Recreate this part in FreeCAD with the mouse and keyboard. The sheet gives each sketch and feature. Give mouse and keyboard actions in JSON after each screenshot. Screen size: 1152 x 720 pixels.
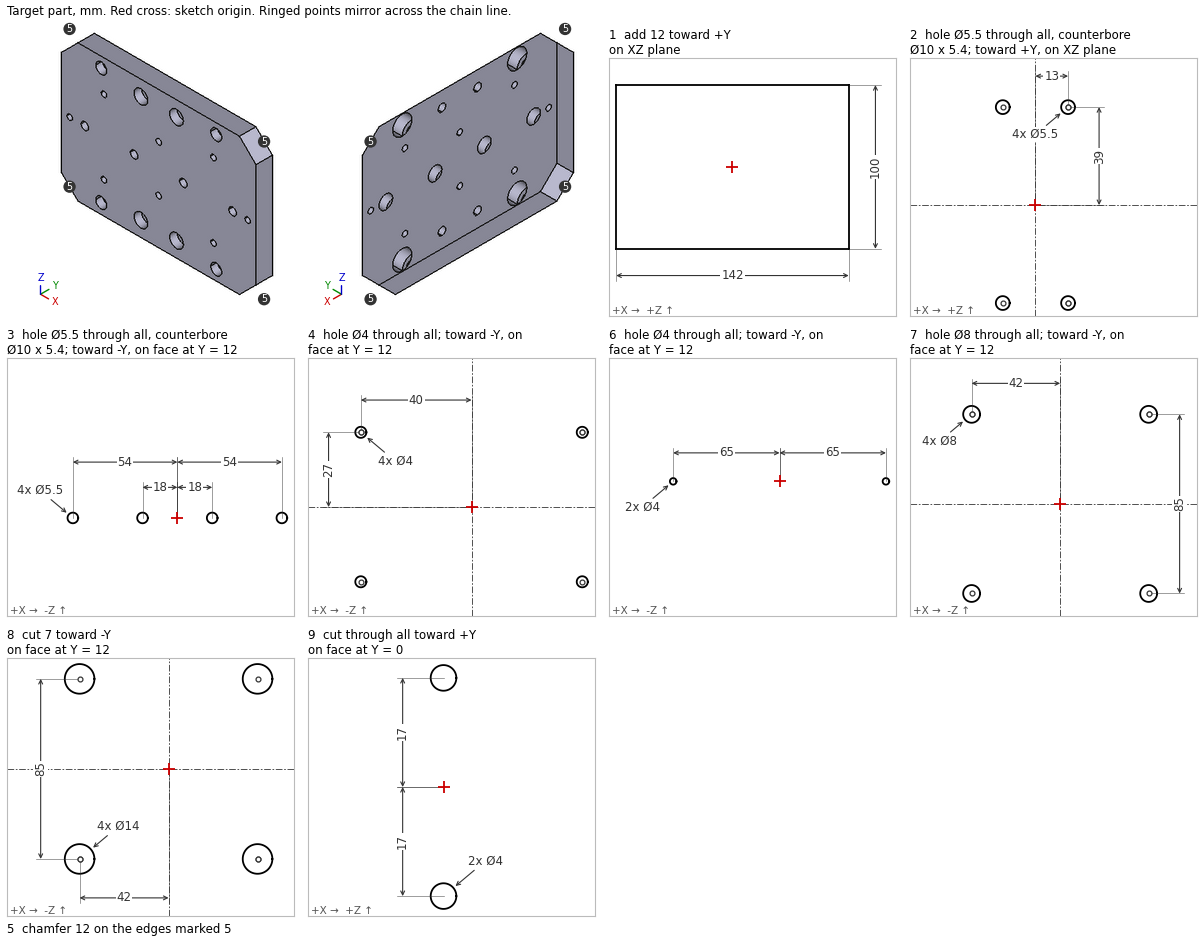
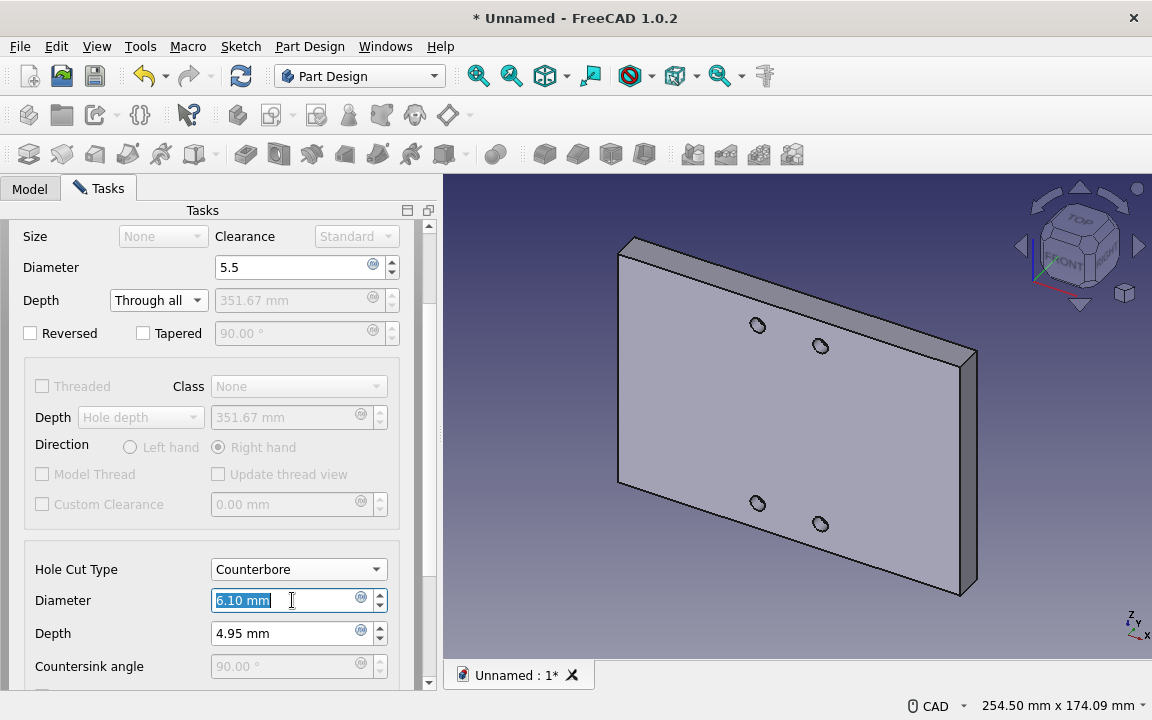
{"action": "type", "text": "10"}
{"action": "key", "text": "Tab"}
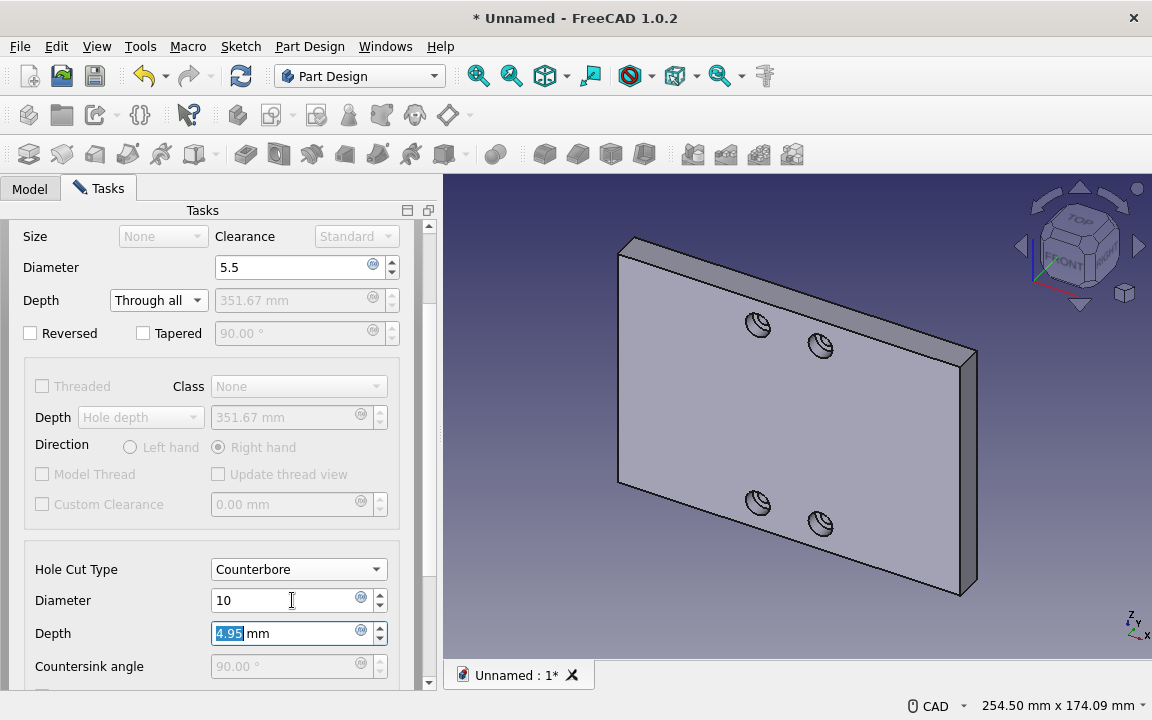
{"action": "type", "text": "5.4"}
{"action": "key", "text": "Tab"}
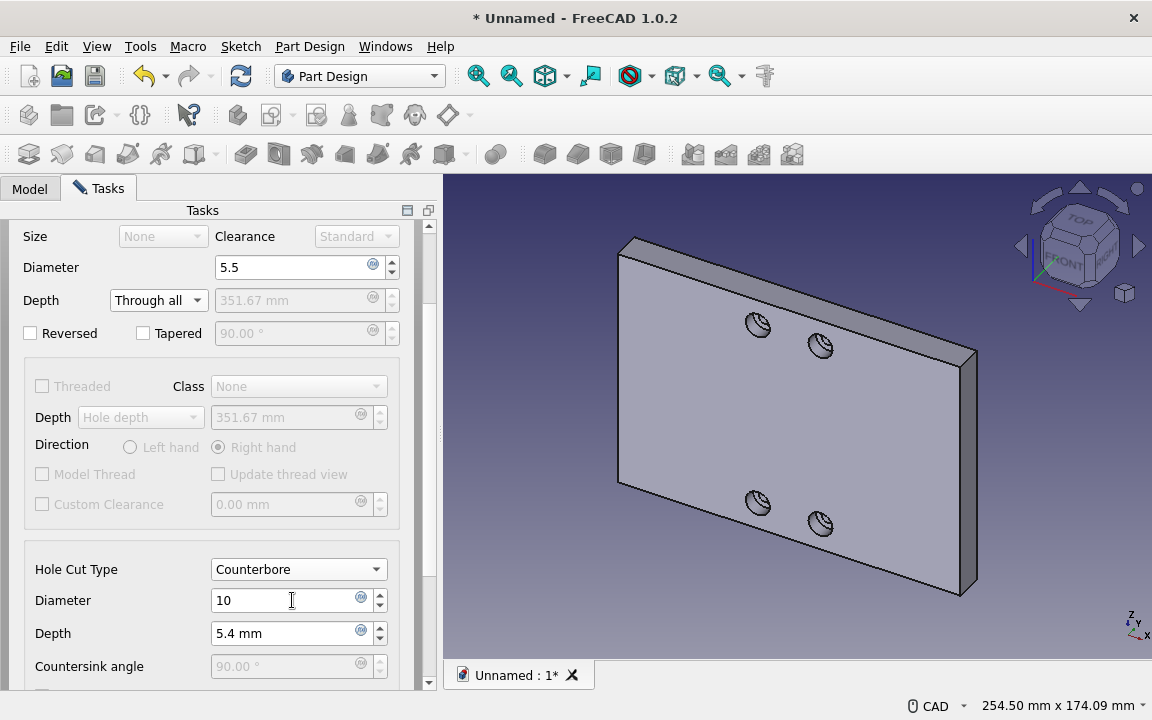
{"action": "scroll", "coordinate": [429, 455], "scroll_direction": "up", "scroll_amount": 3}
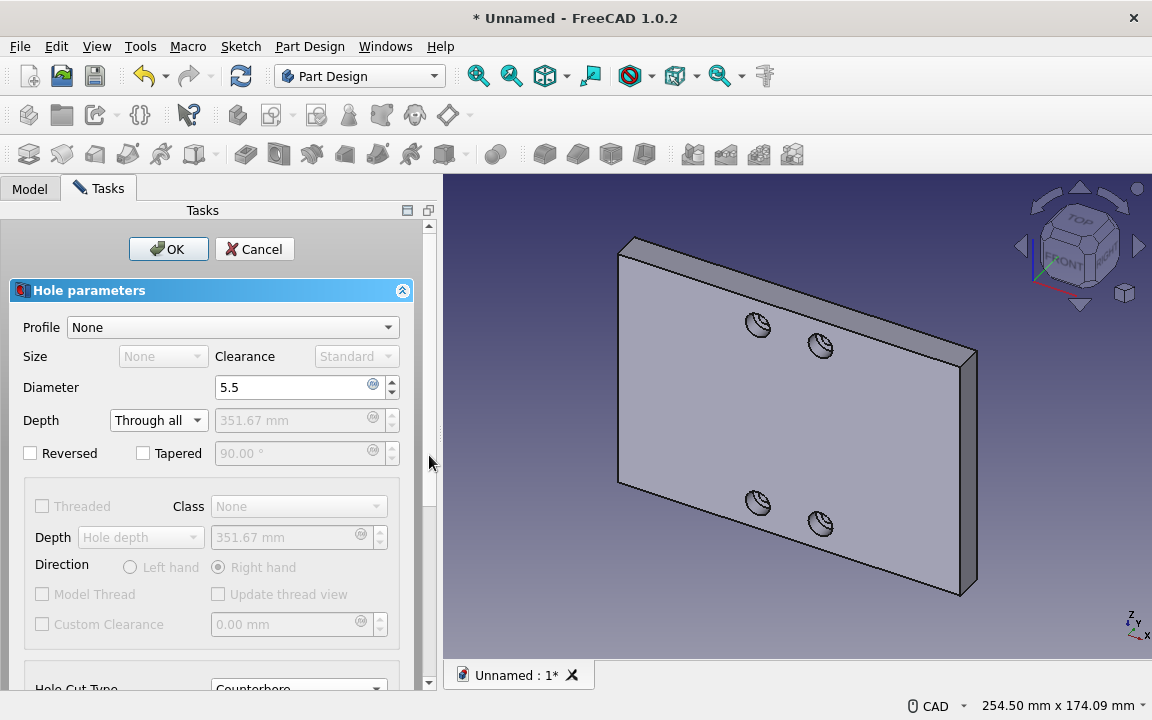
{"action": "left_click", "coordinate": [169, 249]}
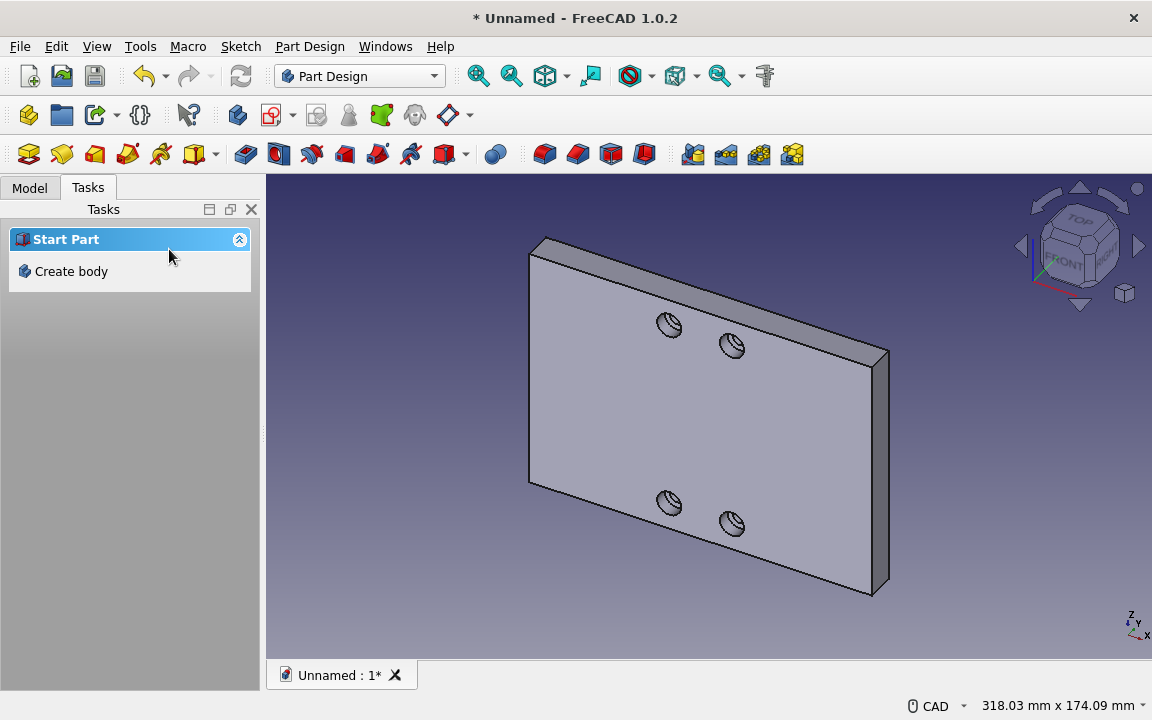
{"action": "key", "text": "4"}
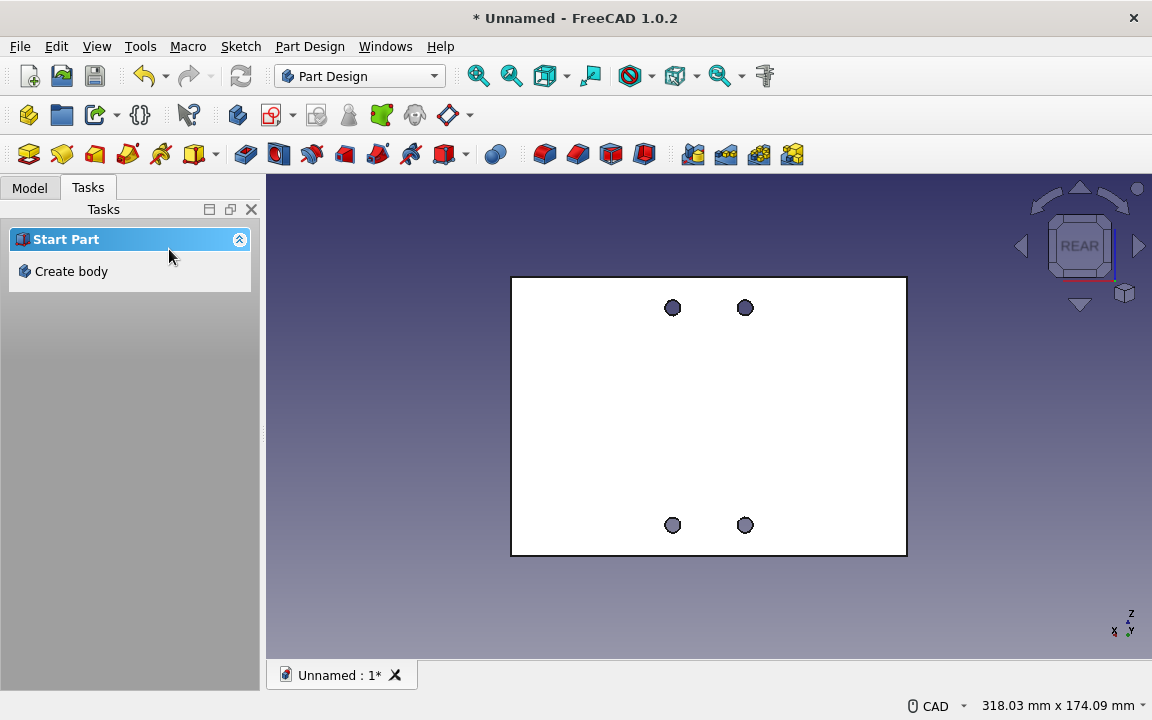
{"action": "left_click", "coordinate": [709, 415]}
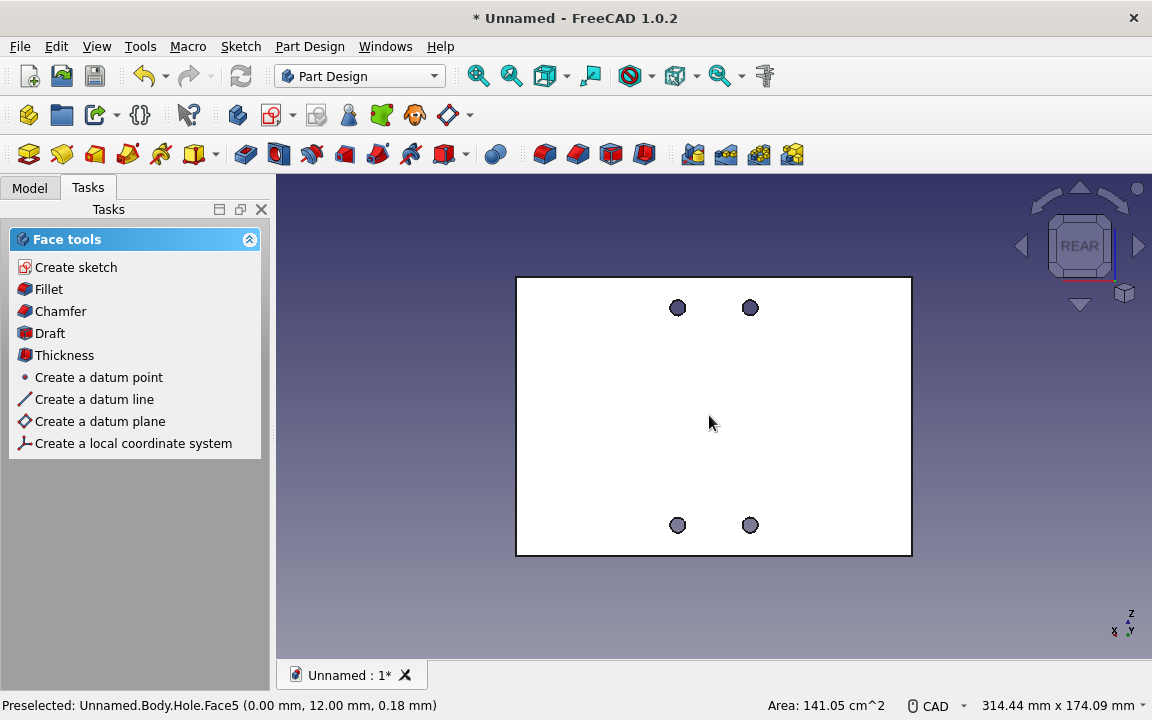
{"action": "left_click", "coordinate": [270, 116]}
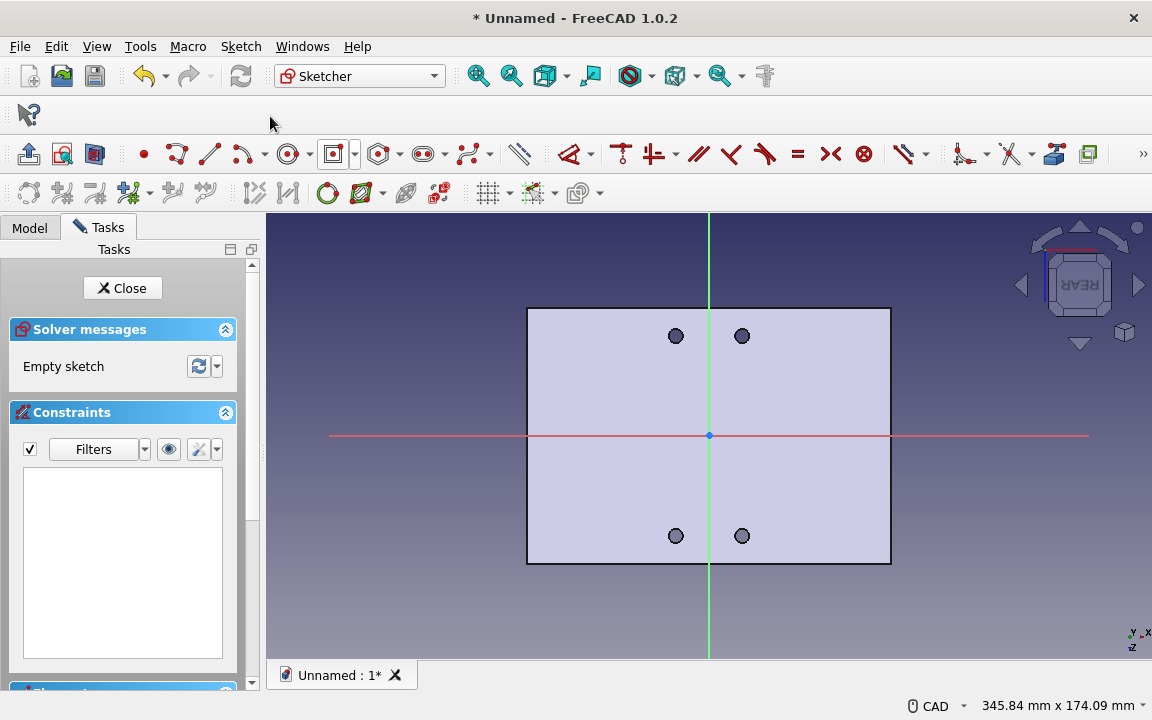
{"action": "scroll", "coordinate": [792, 436], "scroll_direction": "up", "scroll_amount": 3}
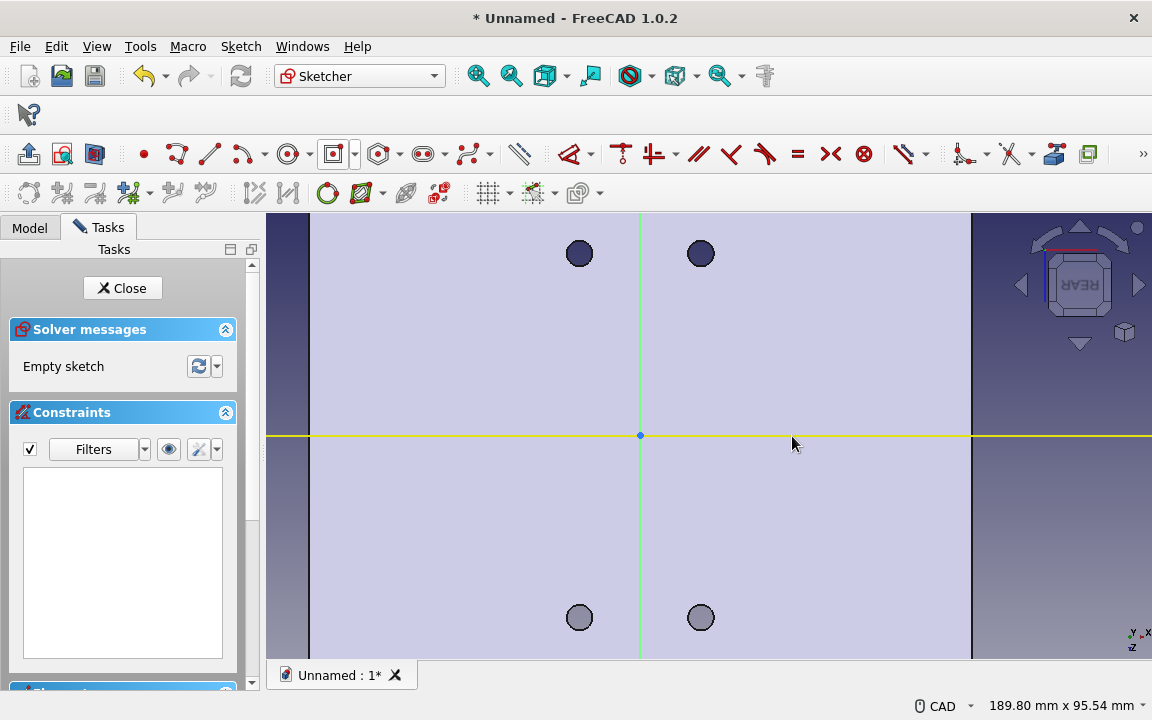
{"action": "left_click", "coordinate": [288, 154]}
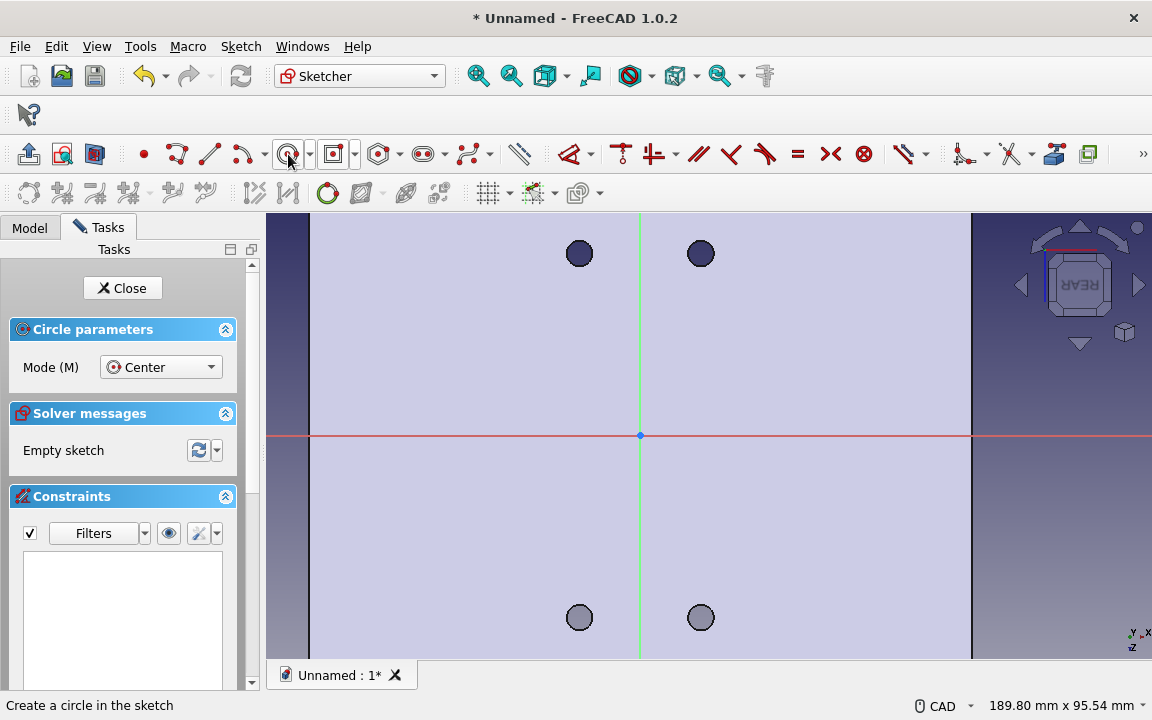
{"action": "scroll", "coordinate": [388, 436], "scroll_direction": "up", "scroll_amount": 3}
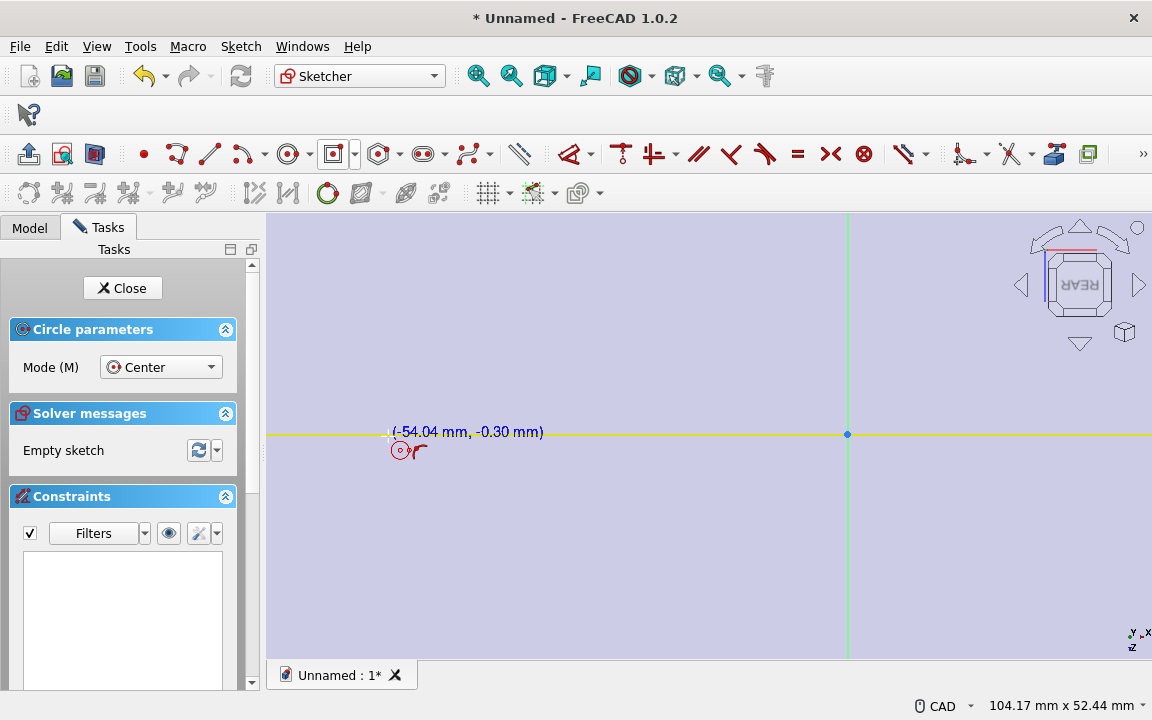
{"action": "left_click", "coordinate": [388, 435]}
{"action": "left_click", "coordinate": [405, 418]}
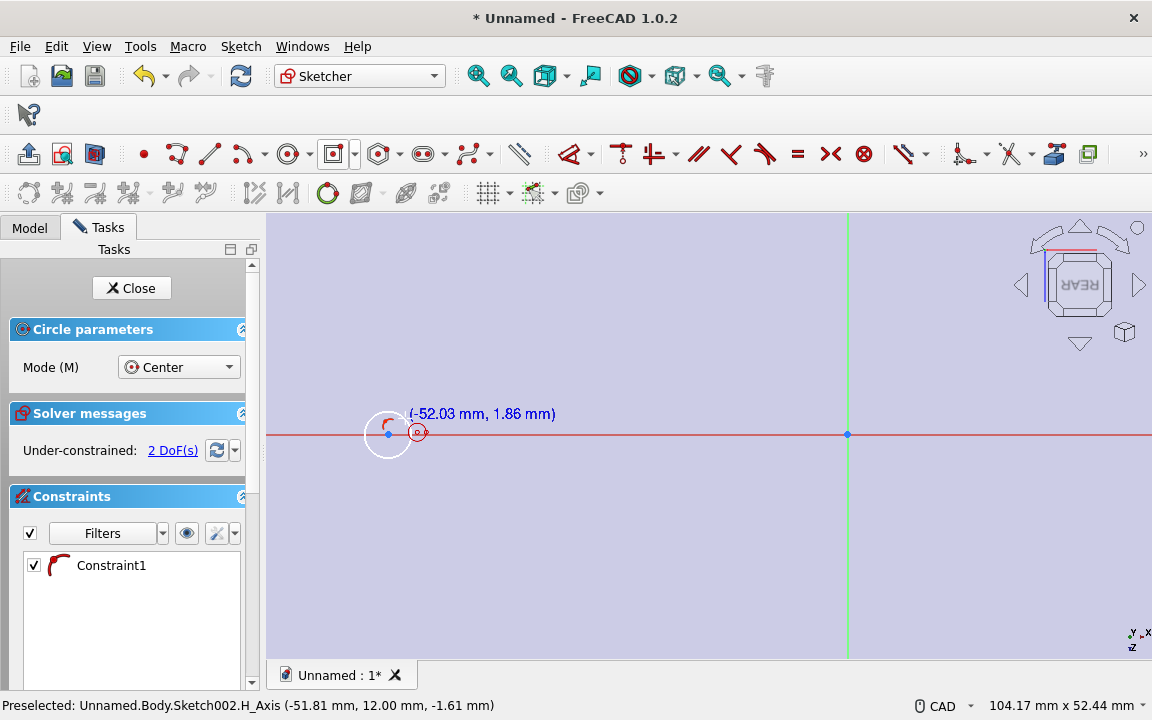
{"action": "scroll", "coordinate": [389, 437], "scroll_direction": "down", "scroll_amount": 3}